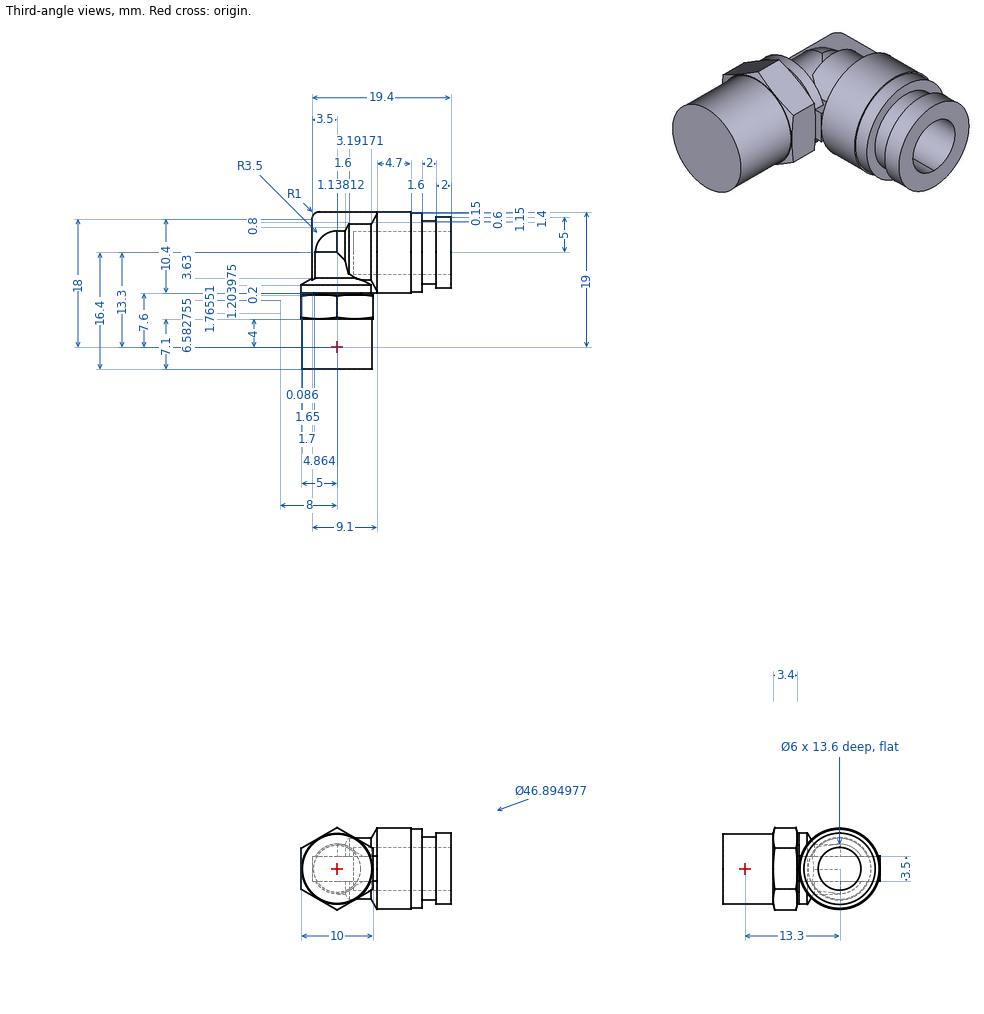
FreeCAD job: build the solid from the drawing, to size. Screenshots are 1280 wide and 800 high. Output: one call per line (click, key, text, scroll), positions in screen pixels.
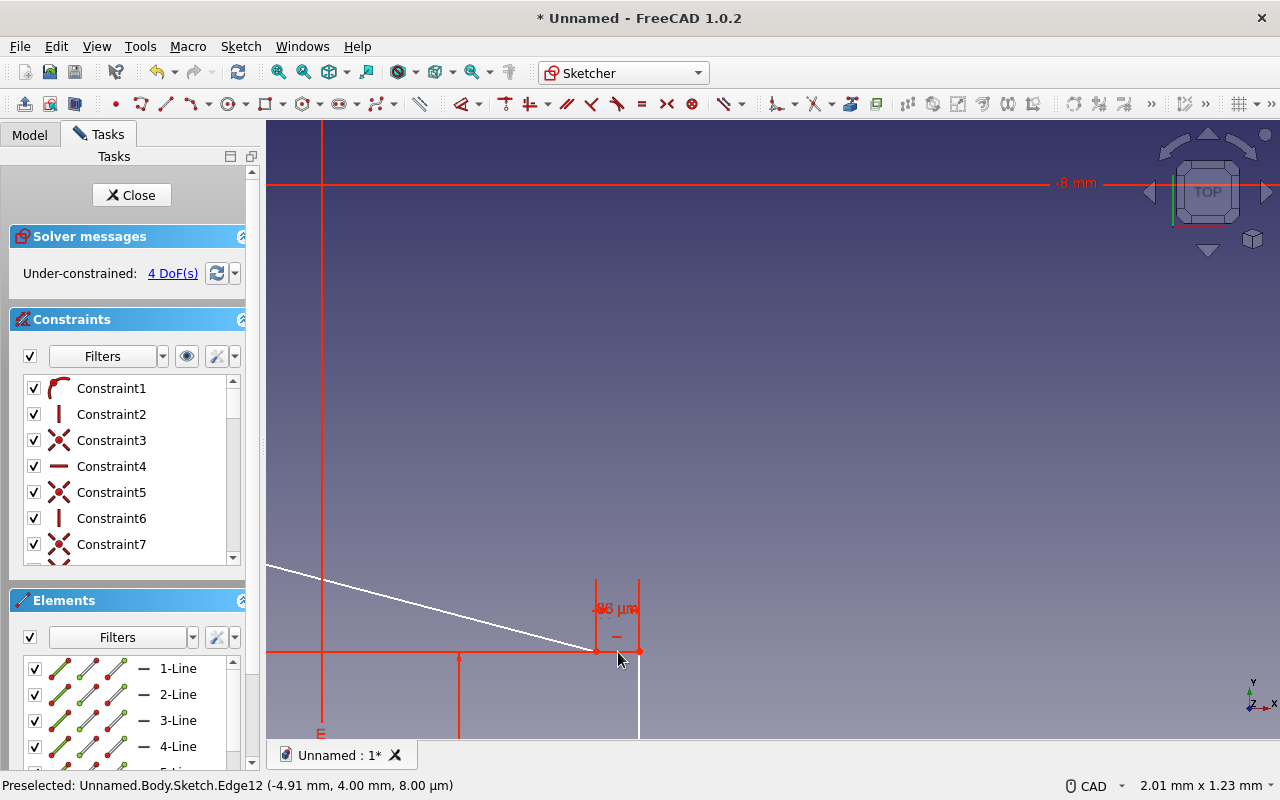
scroll(685, 447, down, 15)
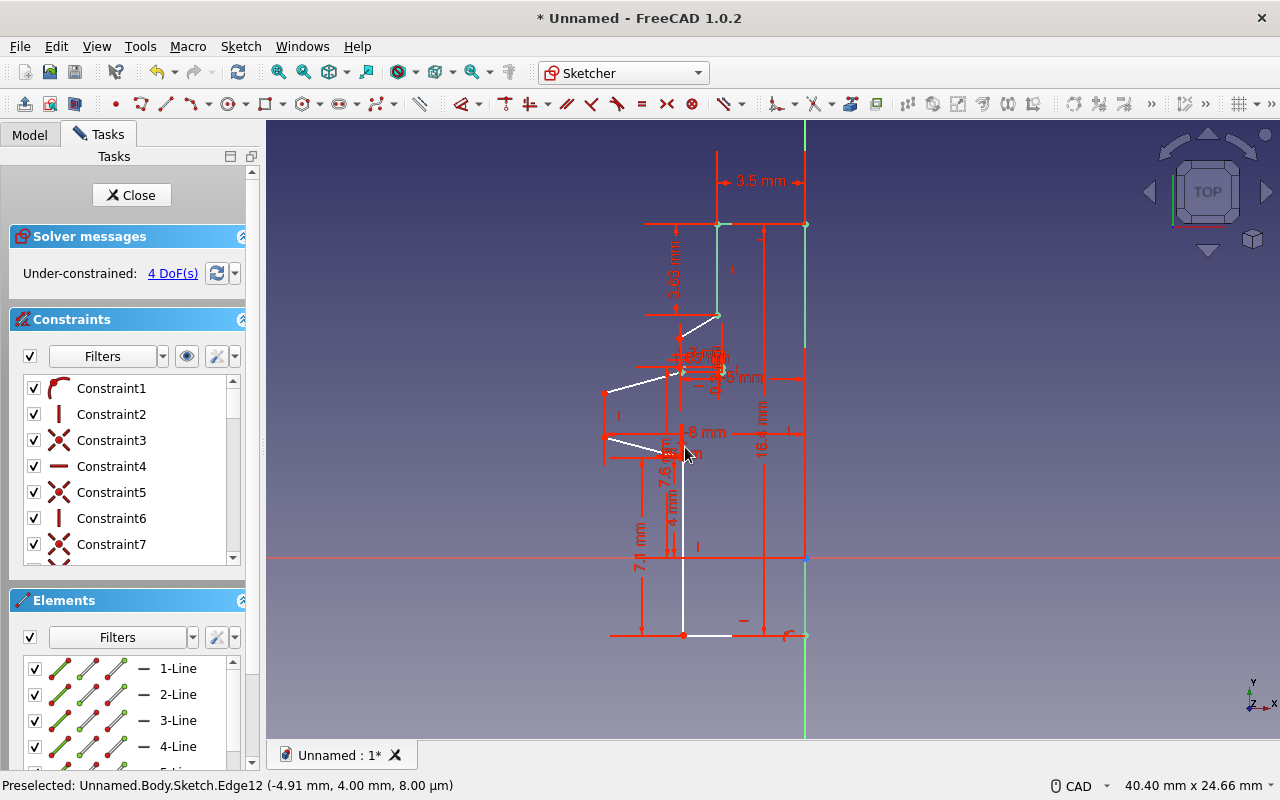
click(720, 636)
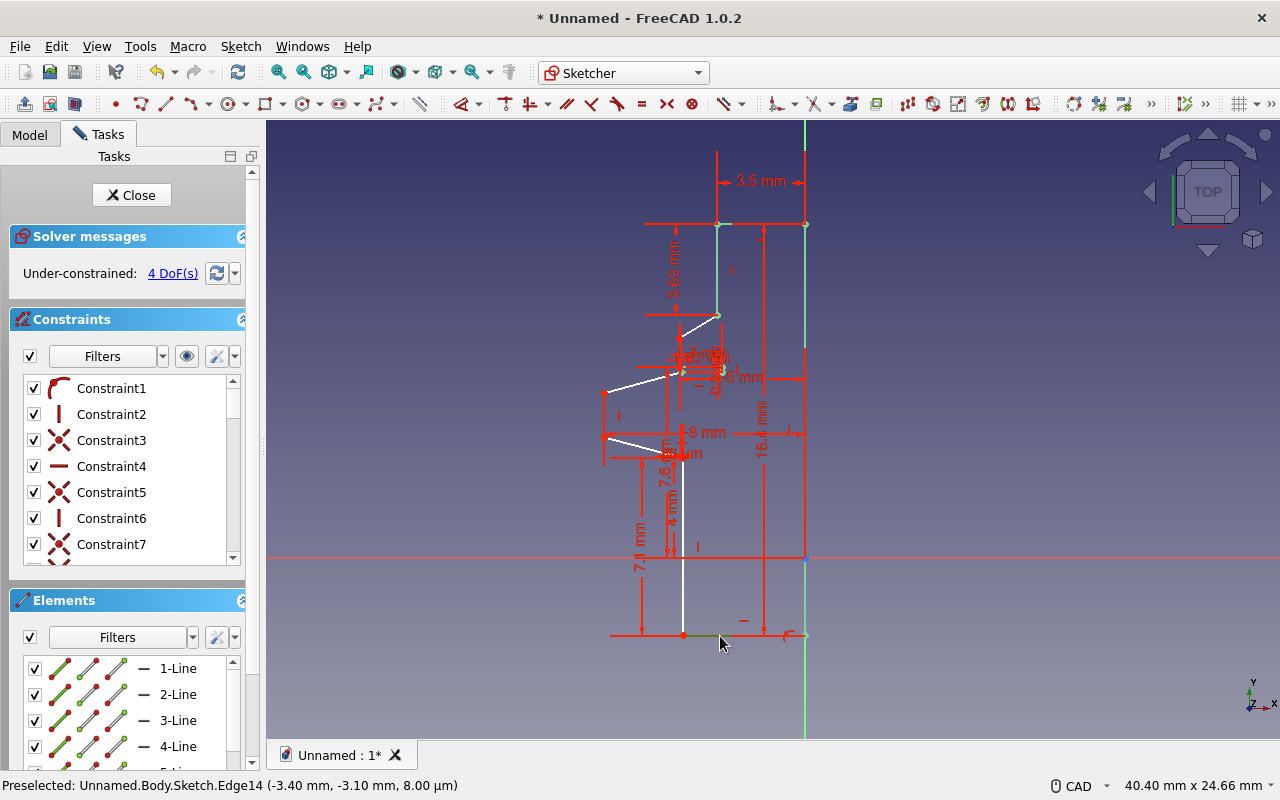
click(478, 104)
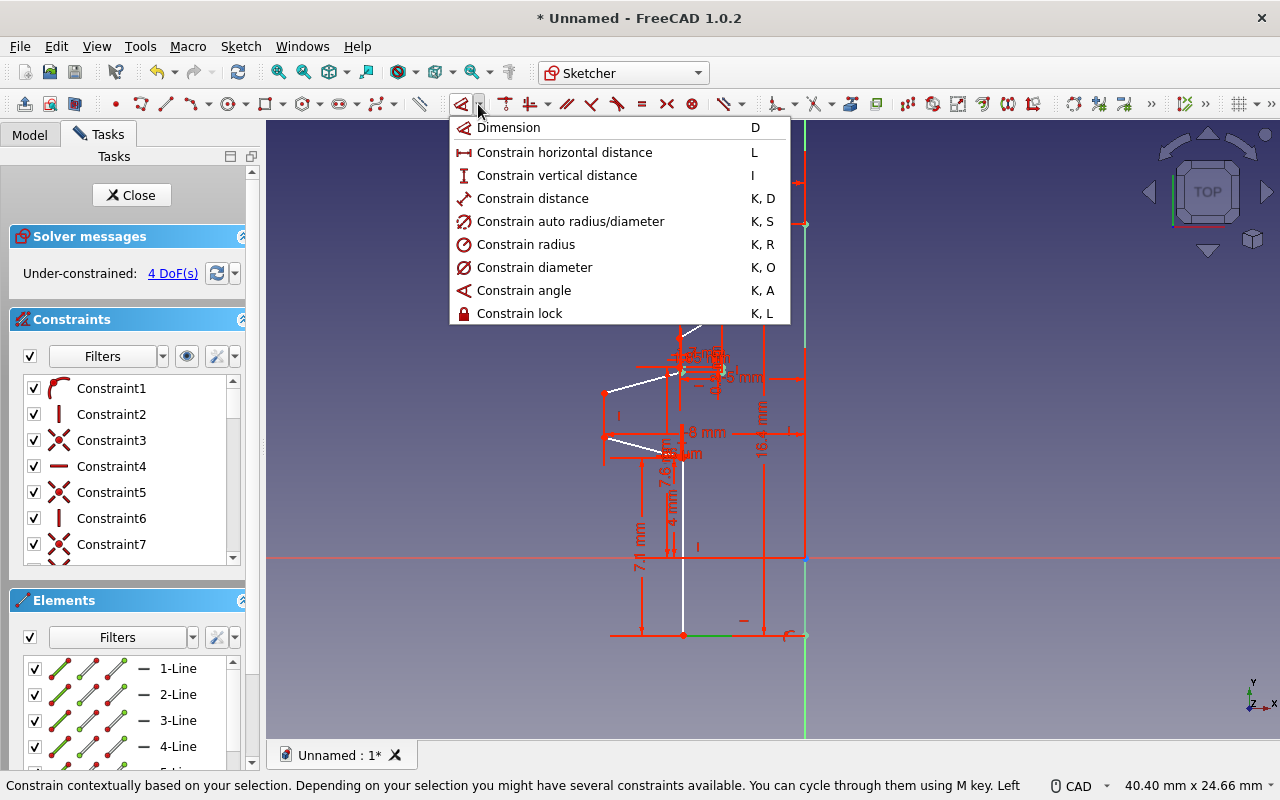
click(620, 152)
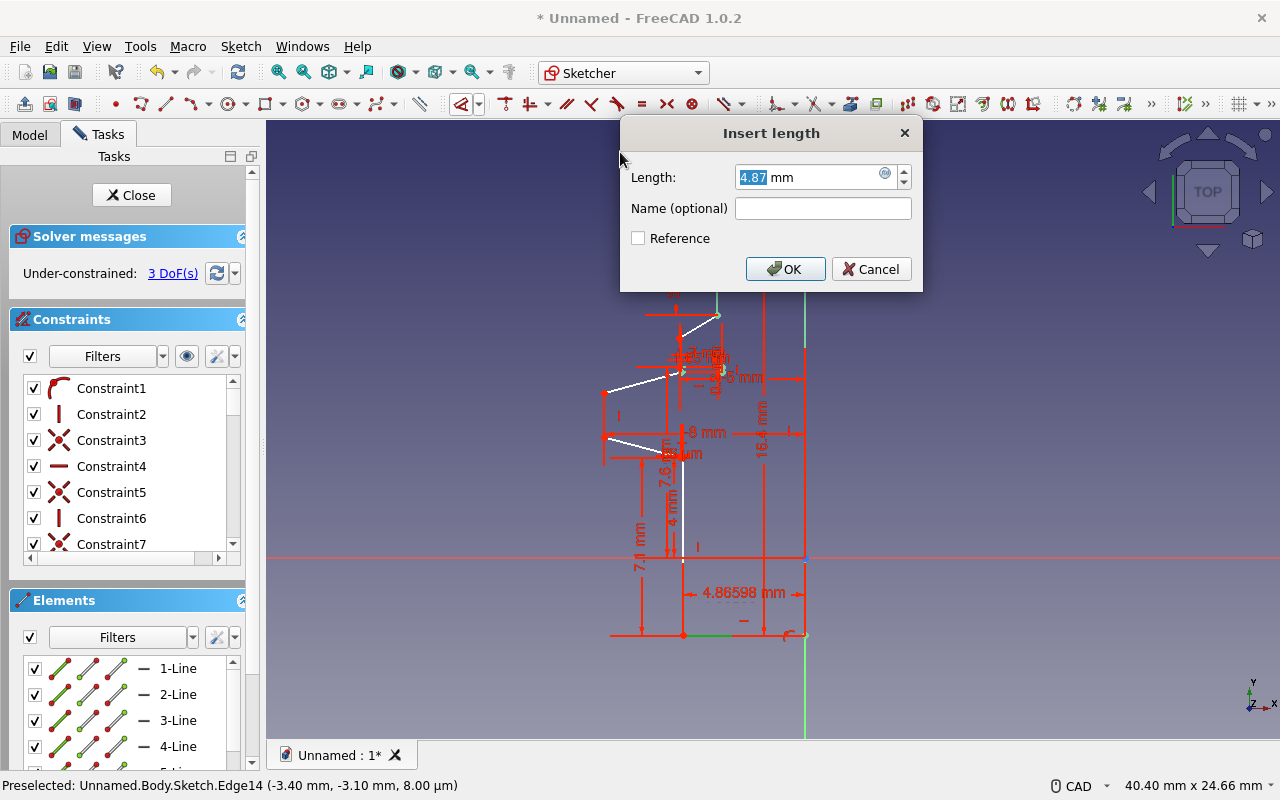
text(4.864)
key(Return)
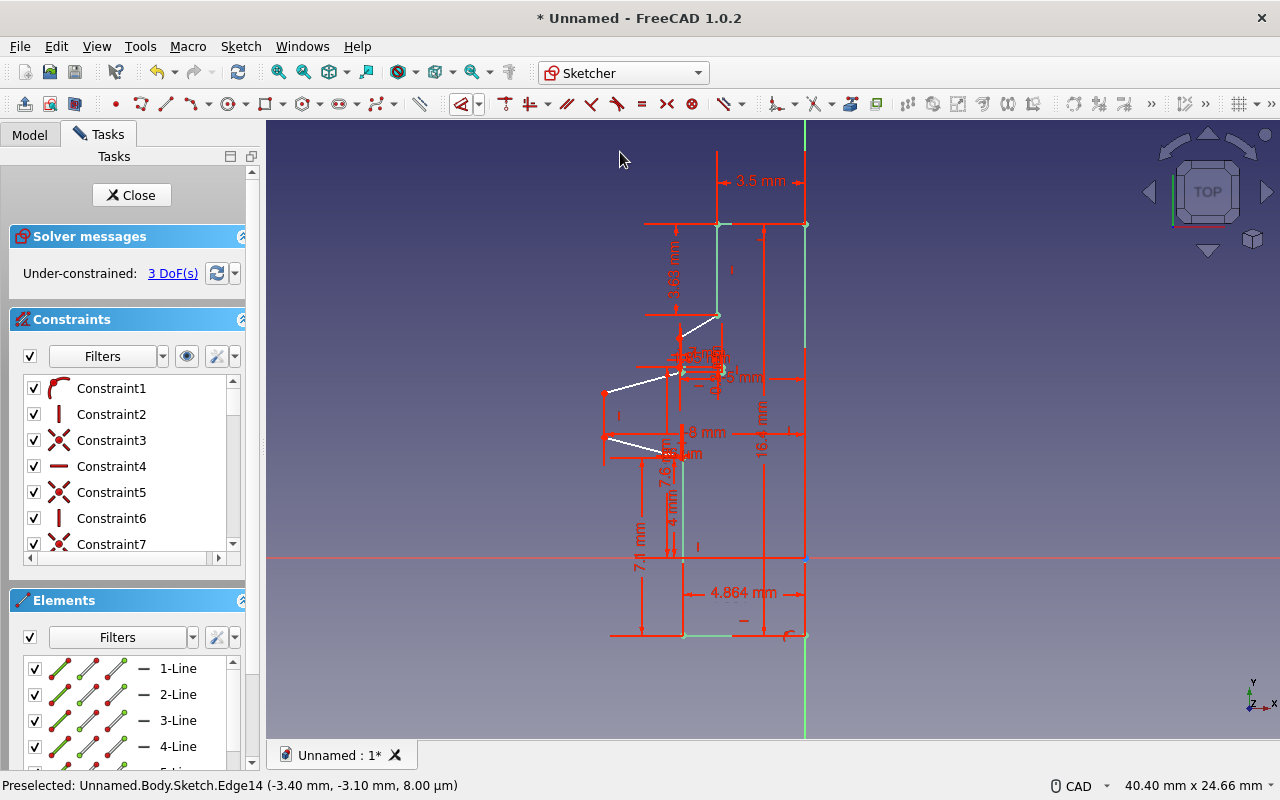
click(604, 406)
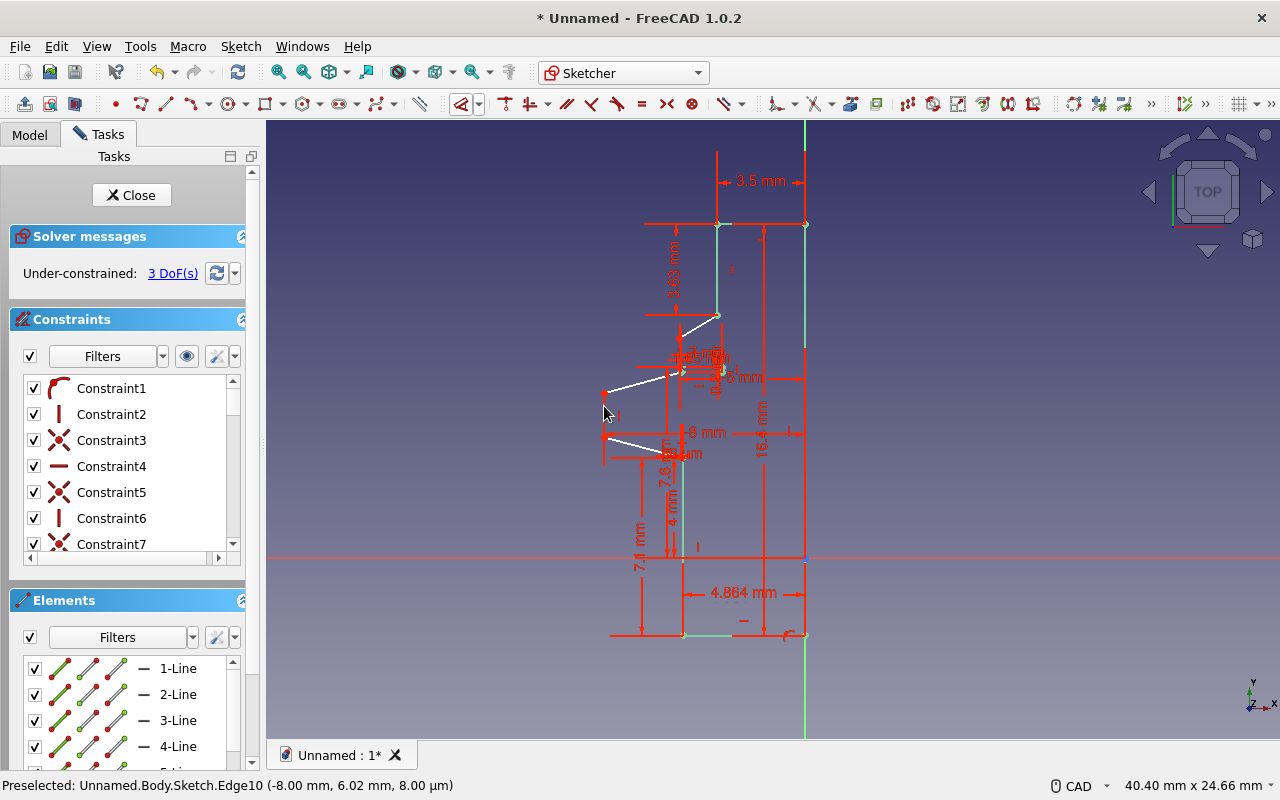
key(i)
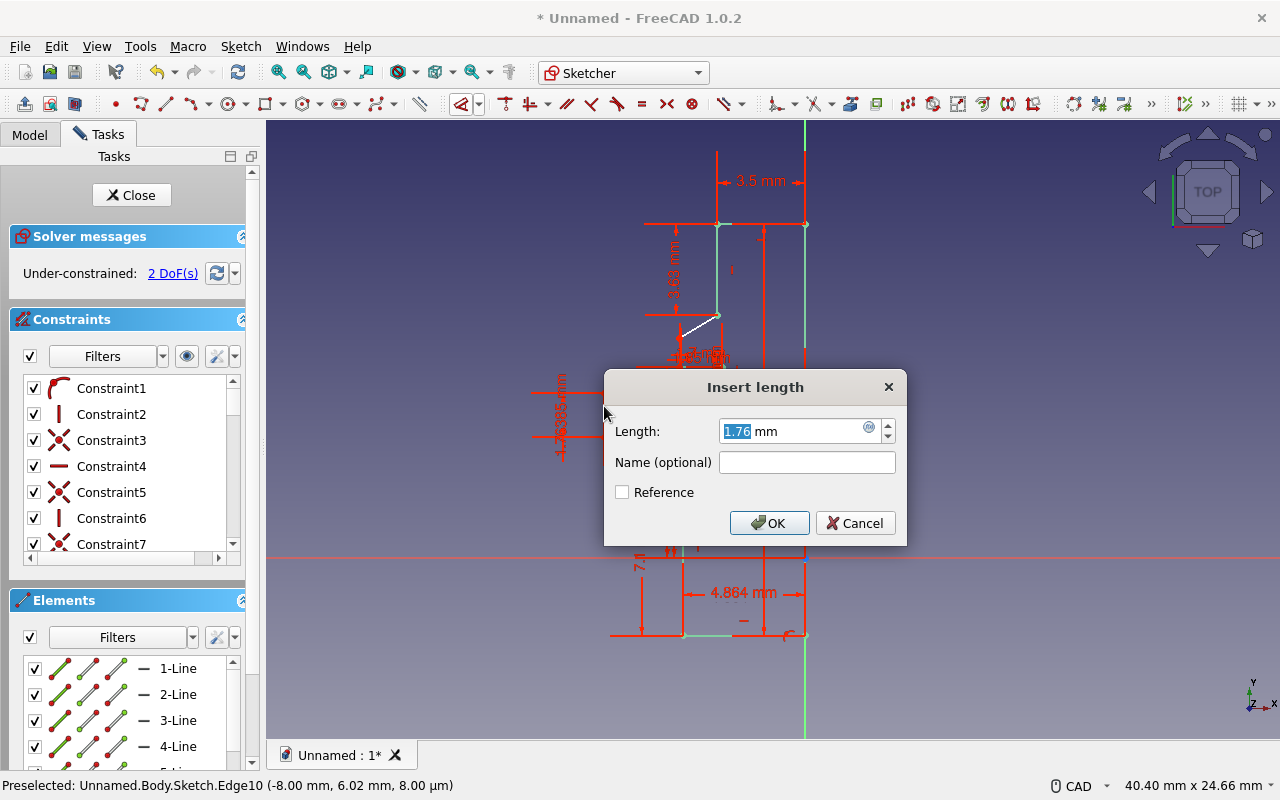
text(1.76551)
key(Return)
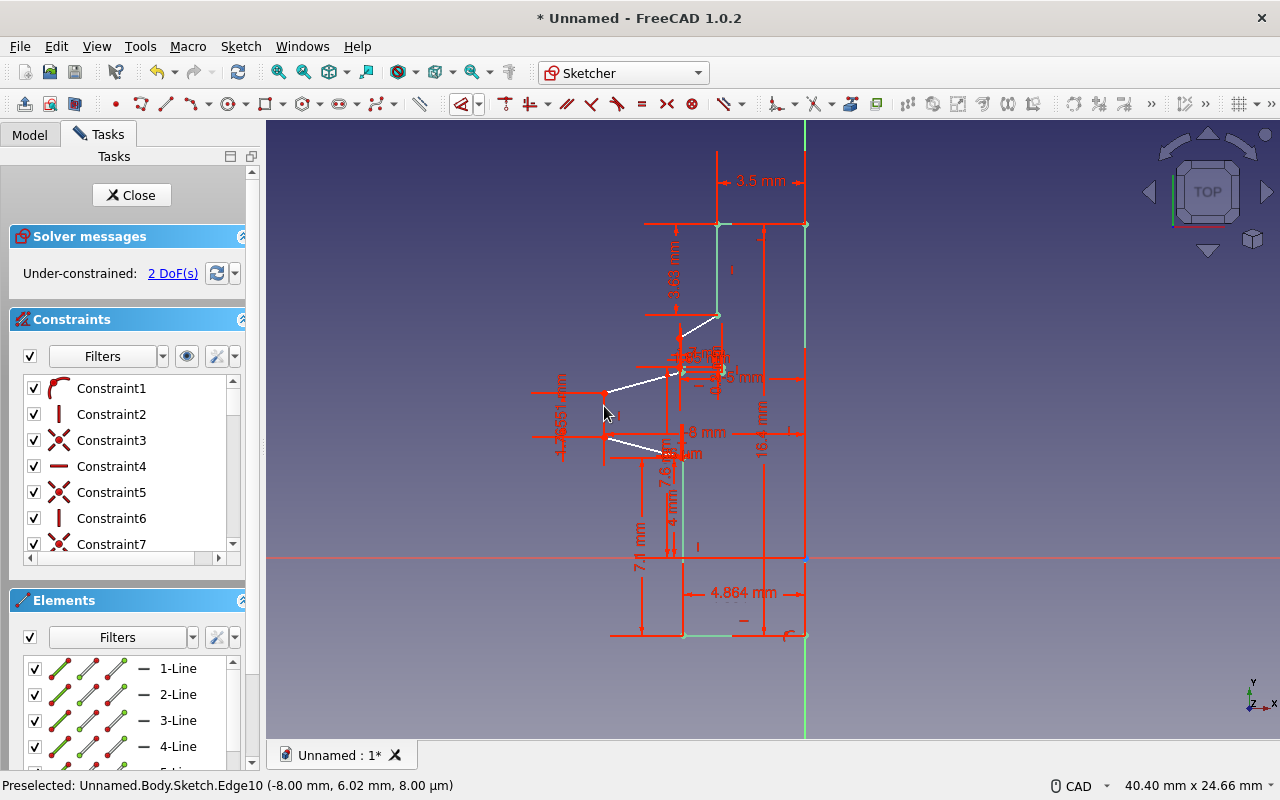
scroll(680, 350, up, 2)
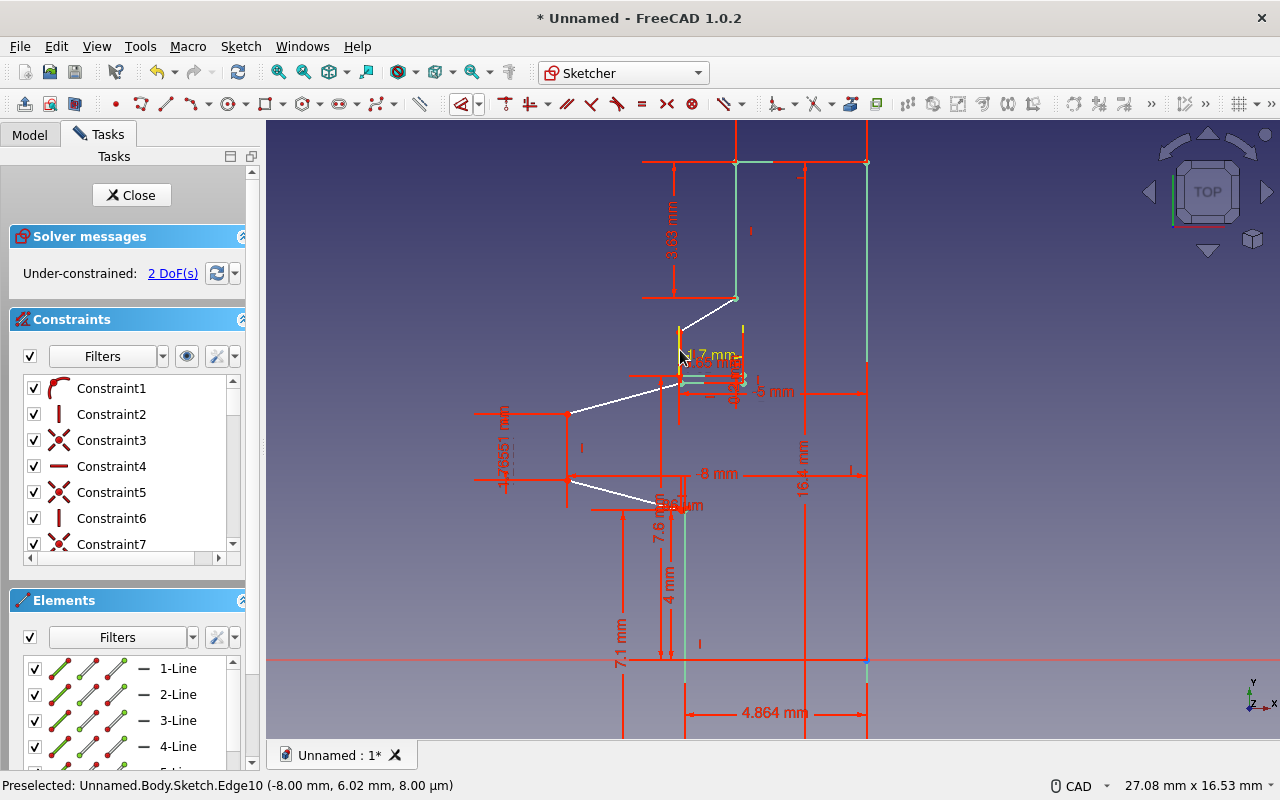
click(679, 350)